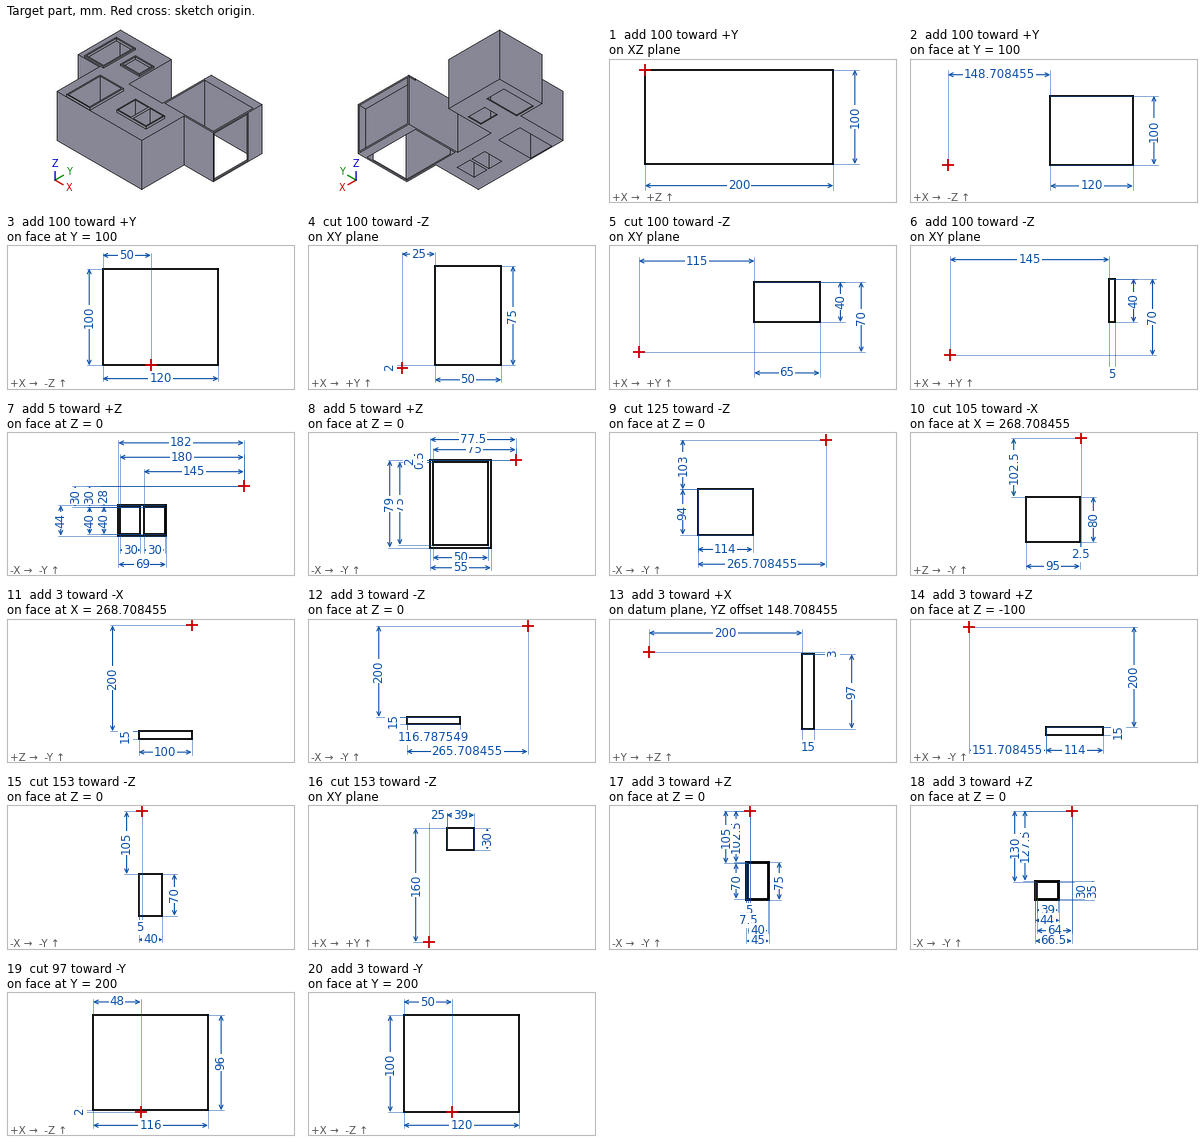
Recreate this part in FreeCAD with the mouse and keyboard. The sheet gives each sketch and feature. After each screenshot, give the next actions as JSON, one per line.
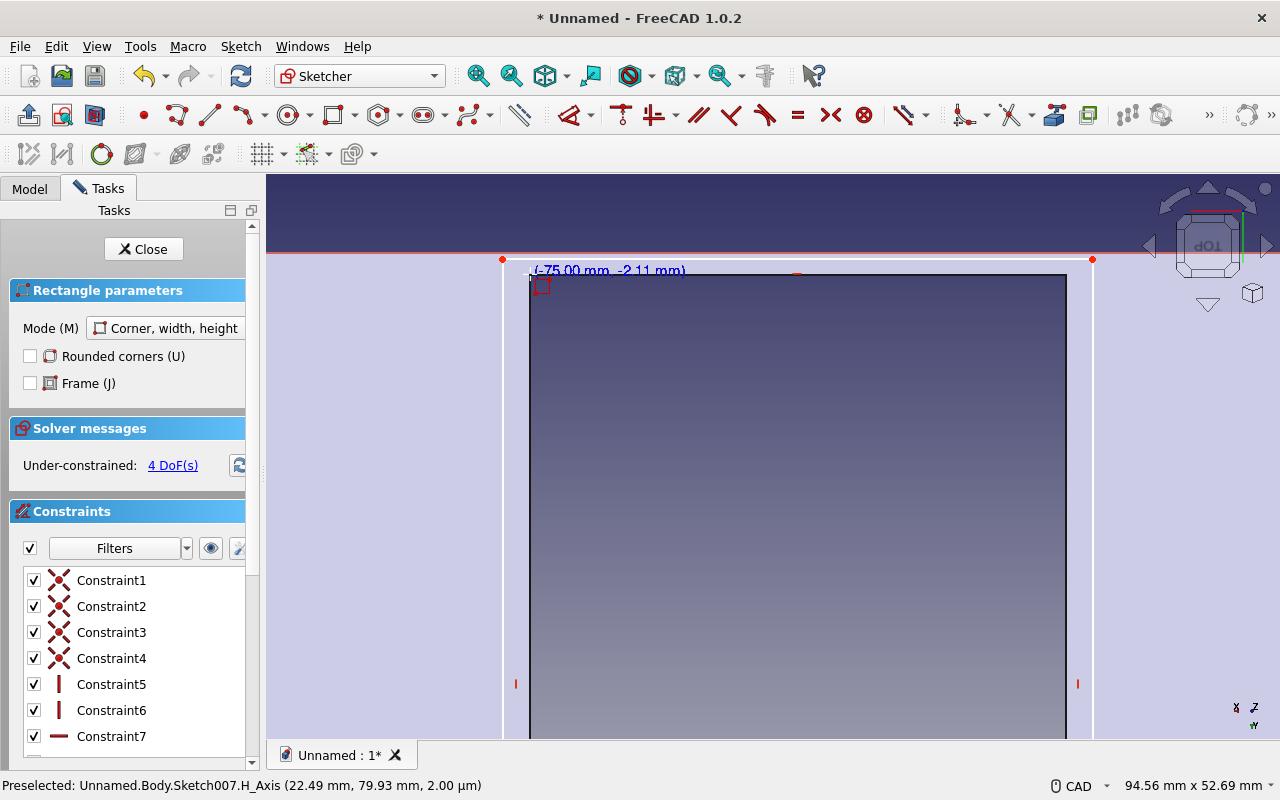
{"action": "left_click", "coordinate": [530, 275]}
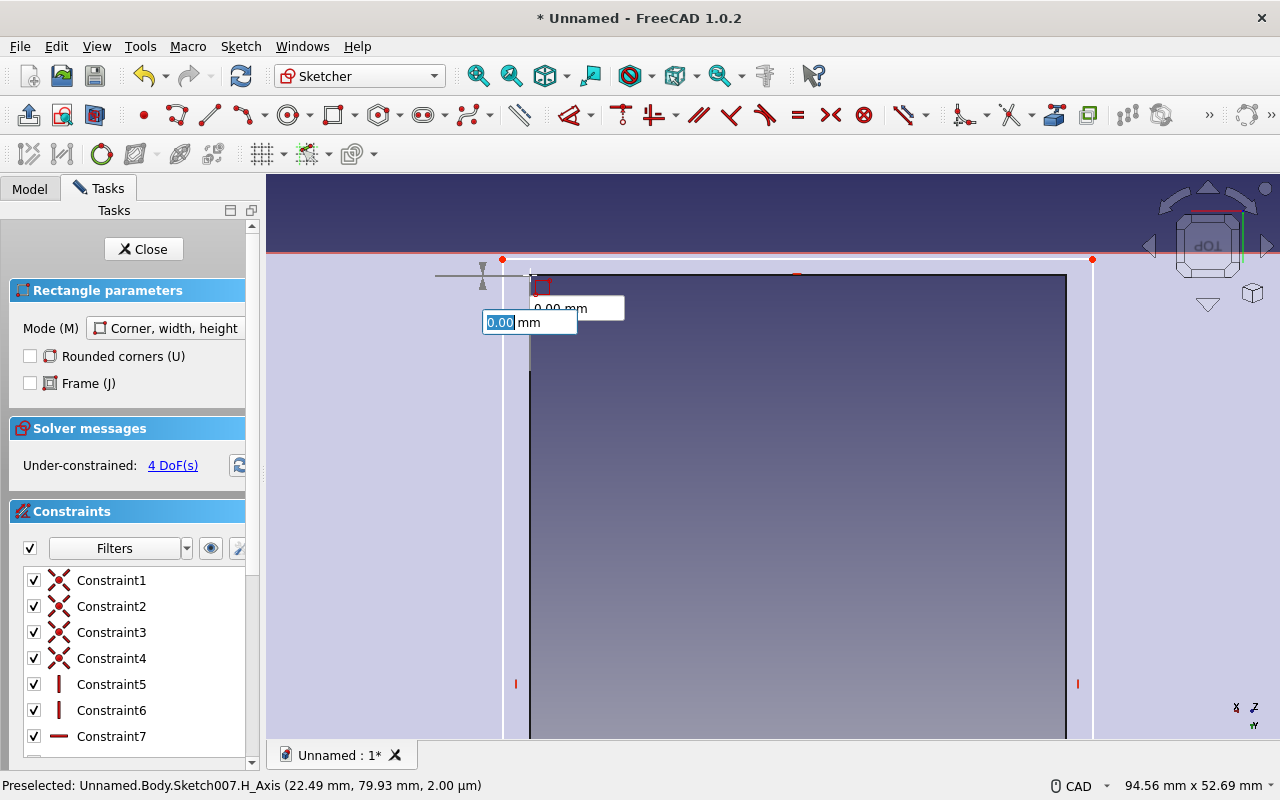
{"action": "scroll", "coordinate": [530, 274], "scroll_direction": "down", "scroll_amount": 4}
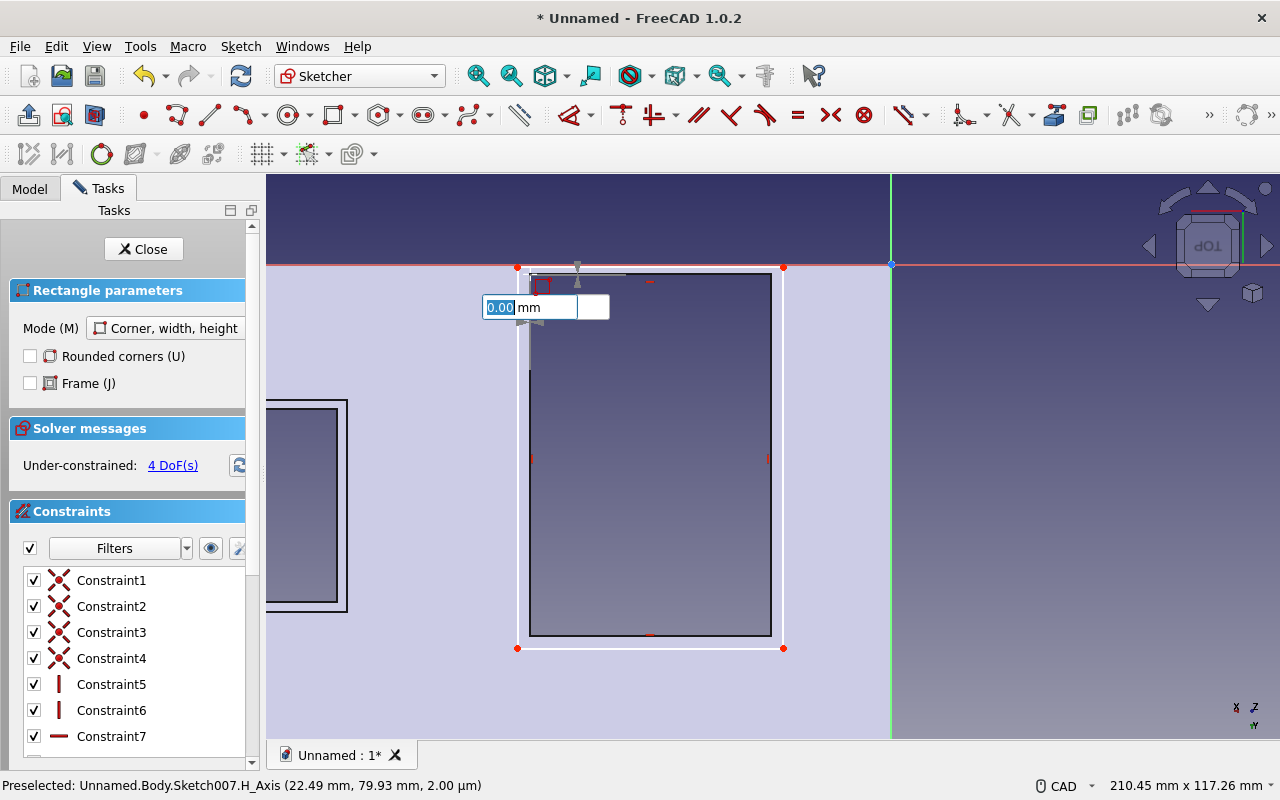
{"action": "scroll", "coordinate": [771, 636], "scroll_direction": "up", "scroll_amount": 2}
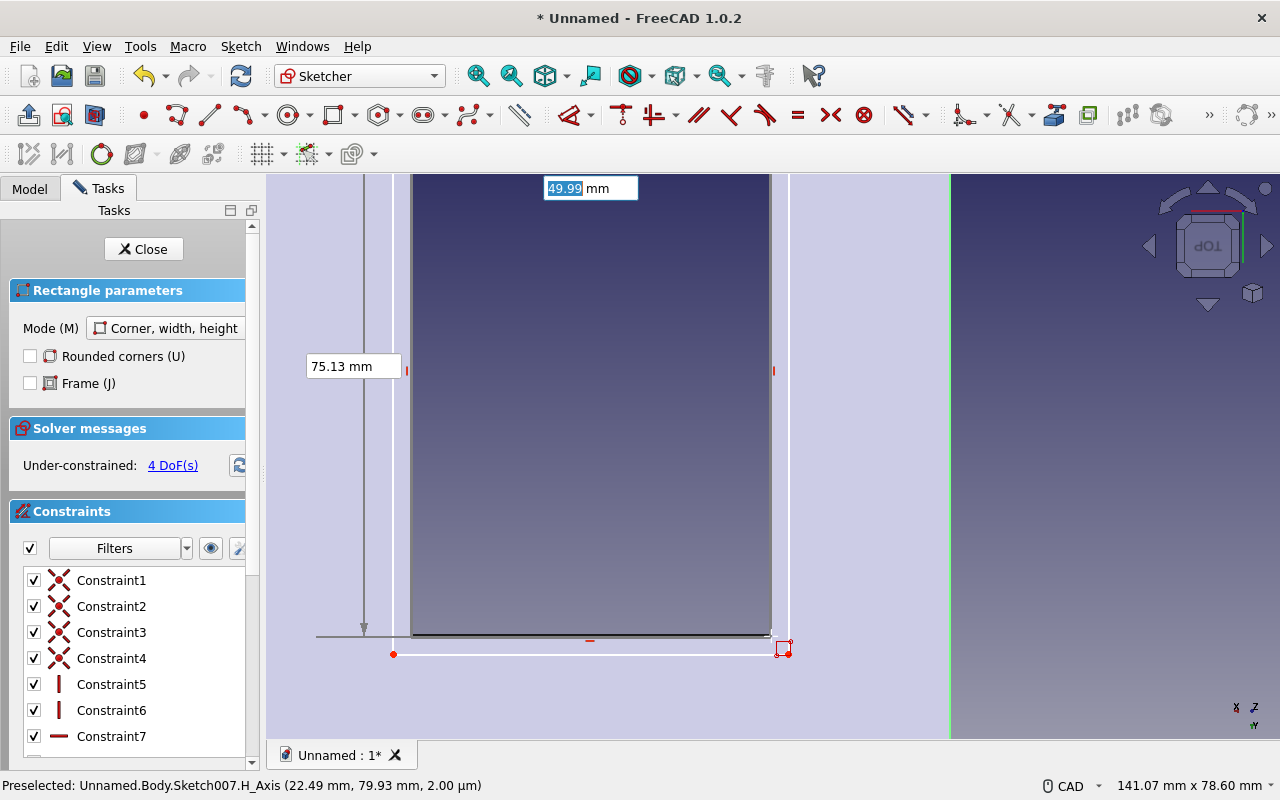
{"action": "left_click", "coordinate": [771, 635]}
{"action": "key", "text": "Escape"}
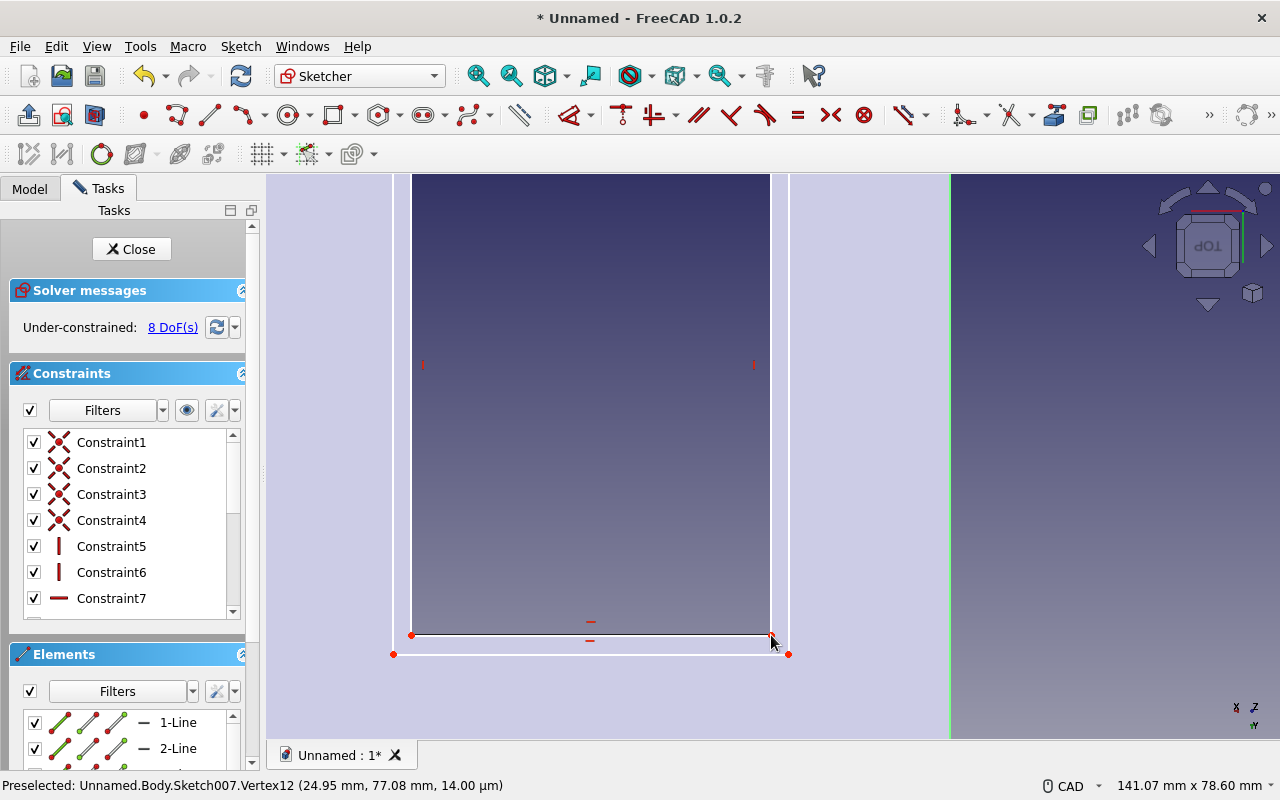
{"action": "left_click", "coordinate": [568, 116]}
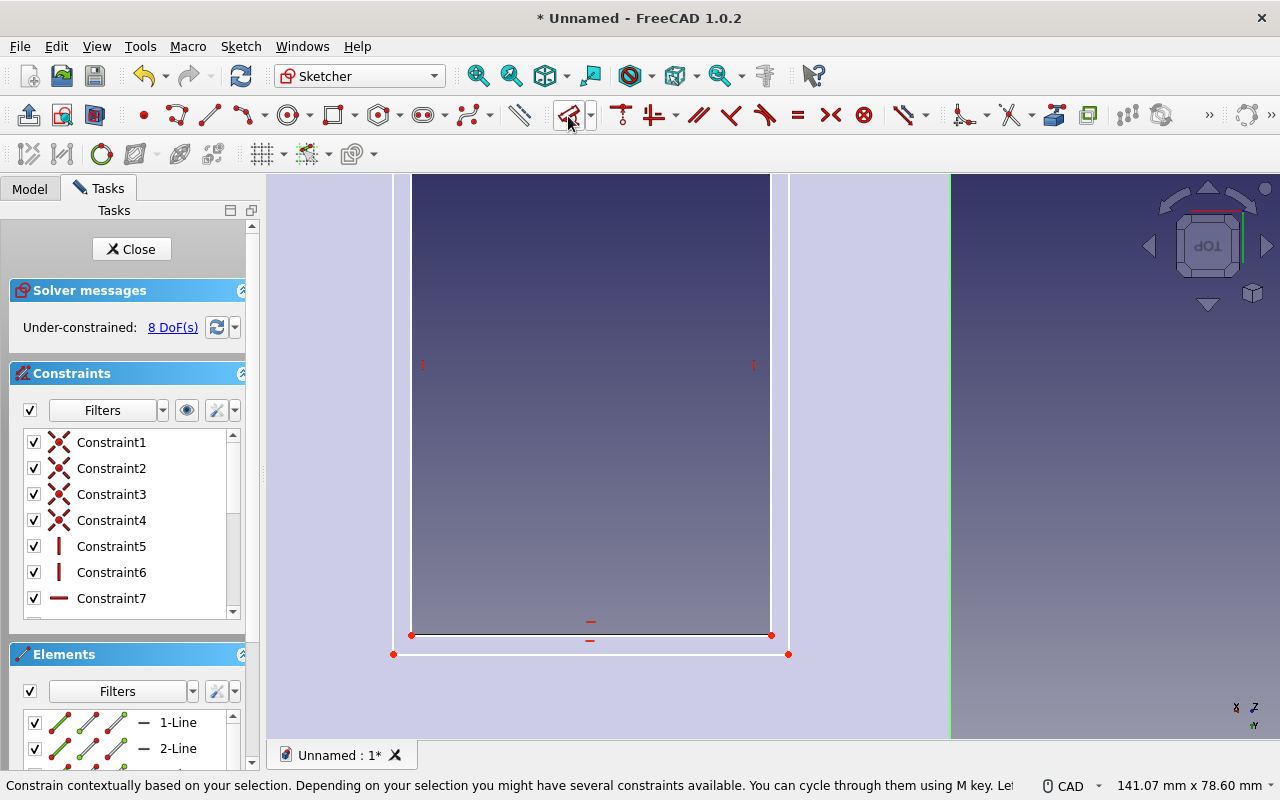
{"action": "left_click", "coordinate": [393, 257]}
{"action": "left_click", "coordinate": [359, 428]}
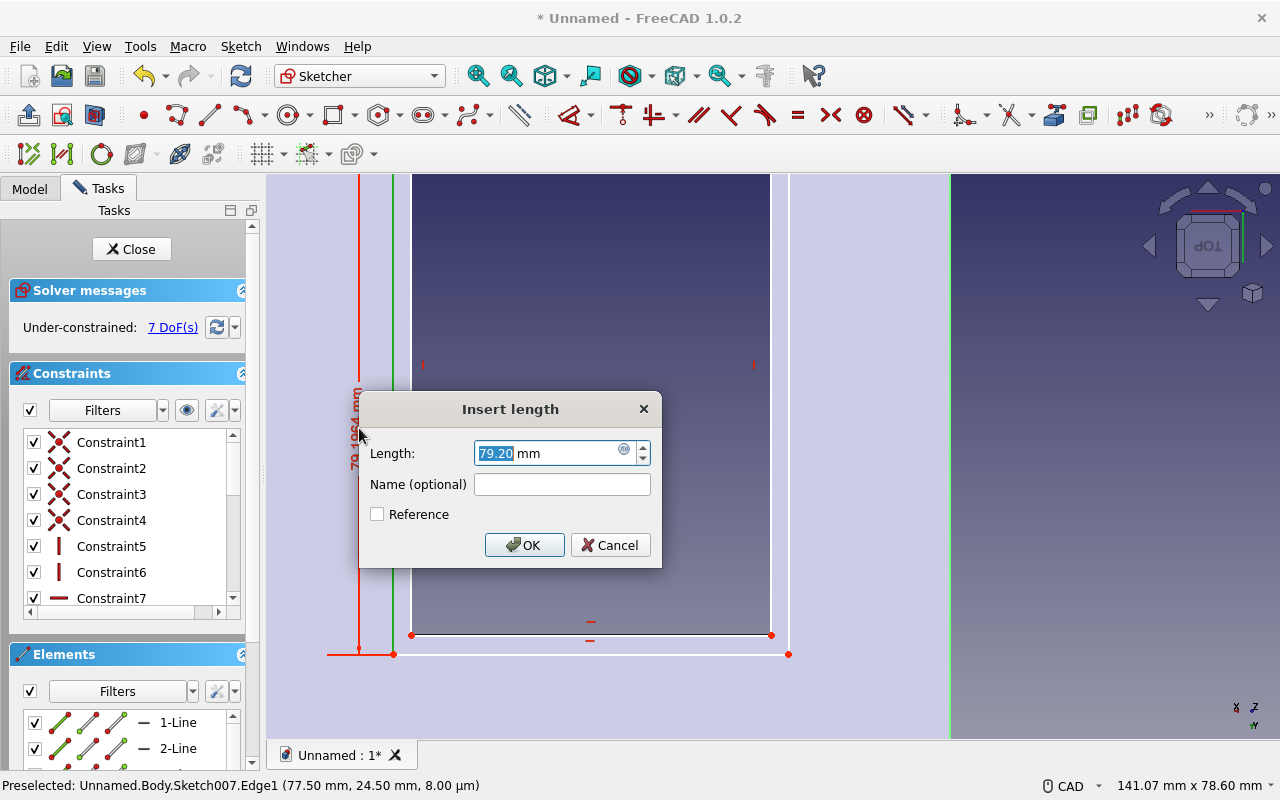
{"action": "type", "text": "79"}
{"action": "key", "text": "Return"}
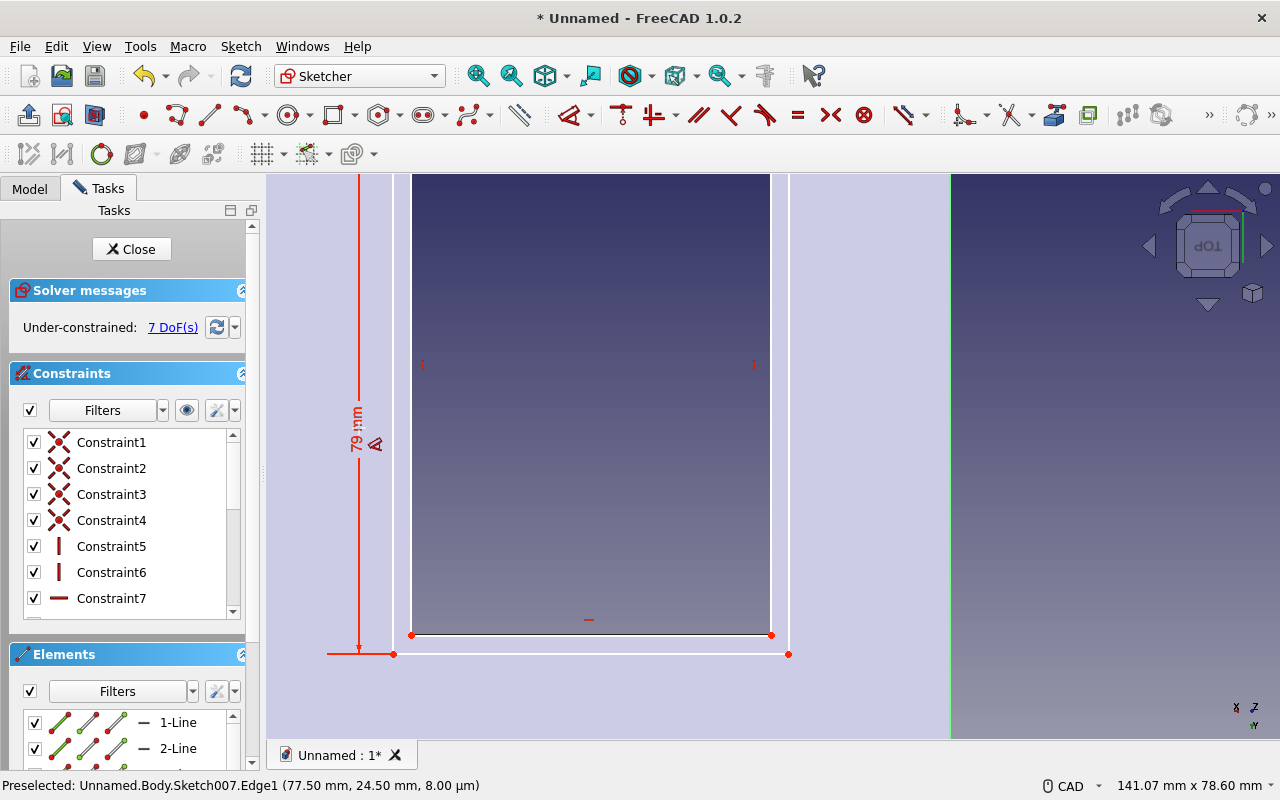
{"action": "left_click", "coordinate": [512, 654]}
{"action": "left_click", "coordinate": [591, 688]}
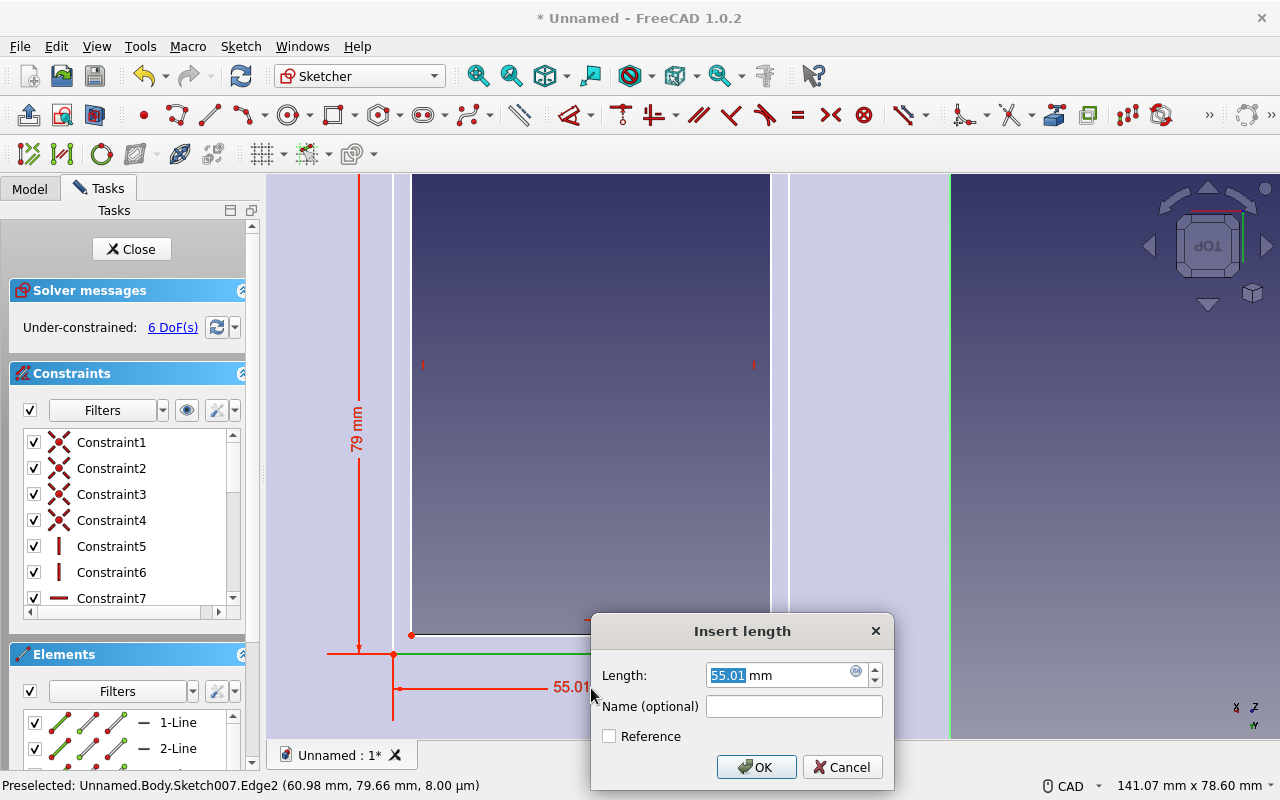
{"action": "type", "text": "55"}
{"action": "key", "text": "Return"}